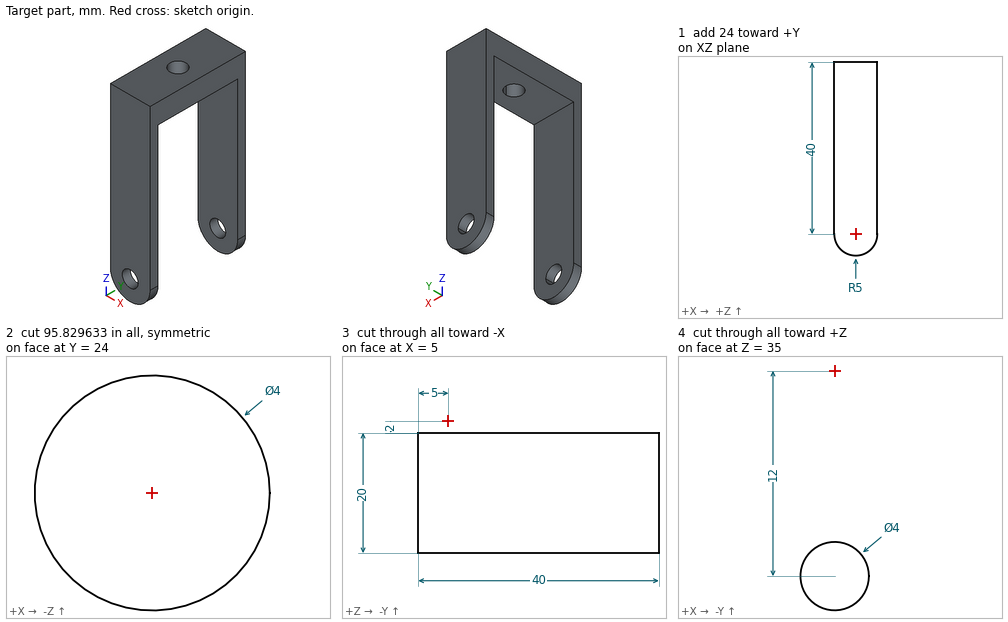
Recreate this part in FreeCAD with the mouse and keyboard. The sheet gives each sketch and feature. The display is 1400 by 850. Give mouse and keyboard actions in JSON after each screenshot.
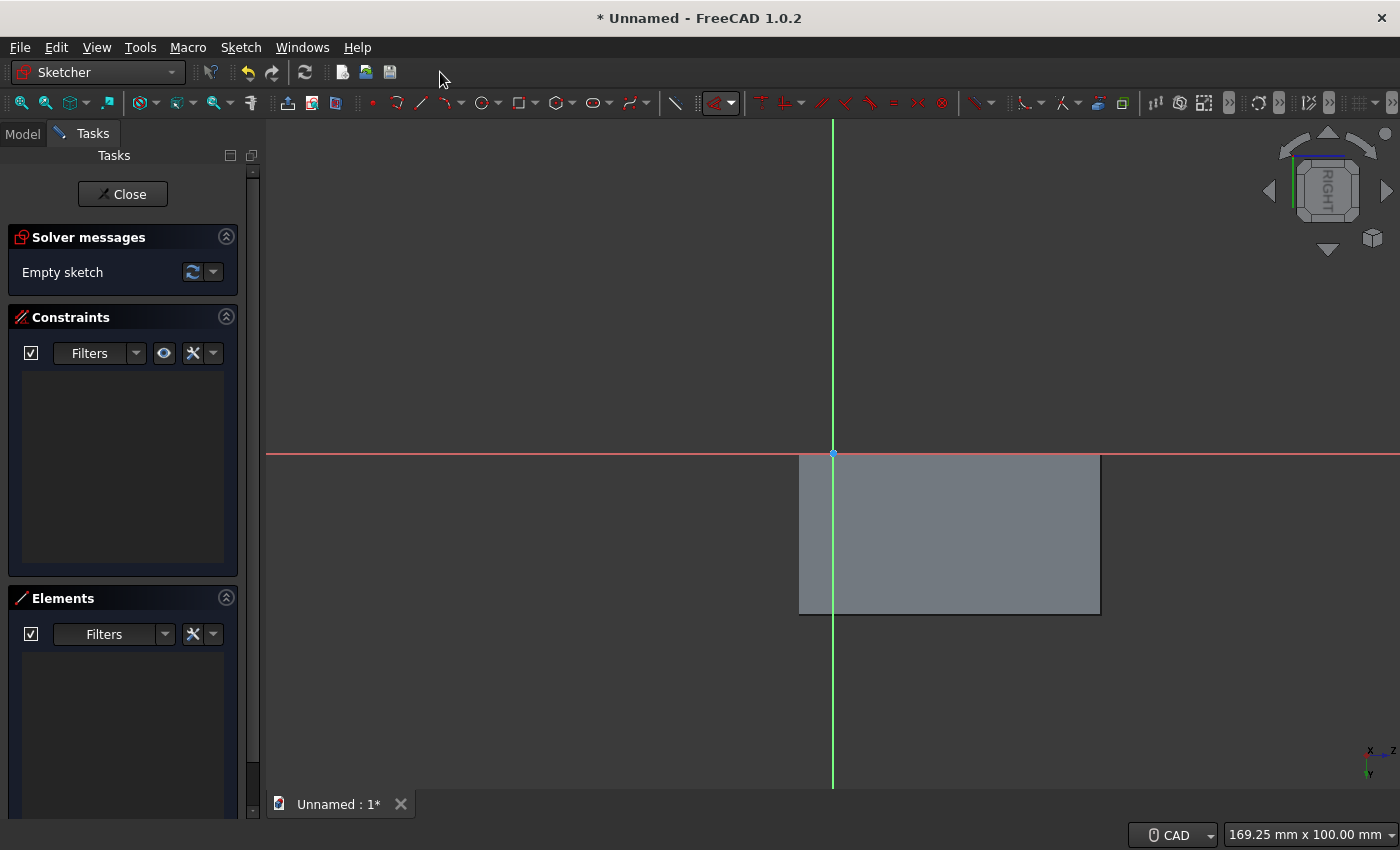
{"action": "scroll", "coordinate": [1032, 571], "scroll_direction": "up", "scroll_amount": 5}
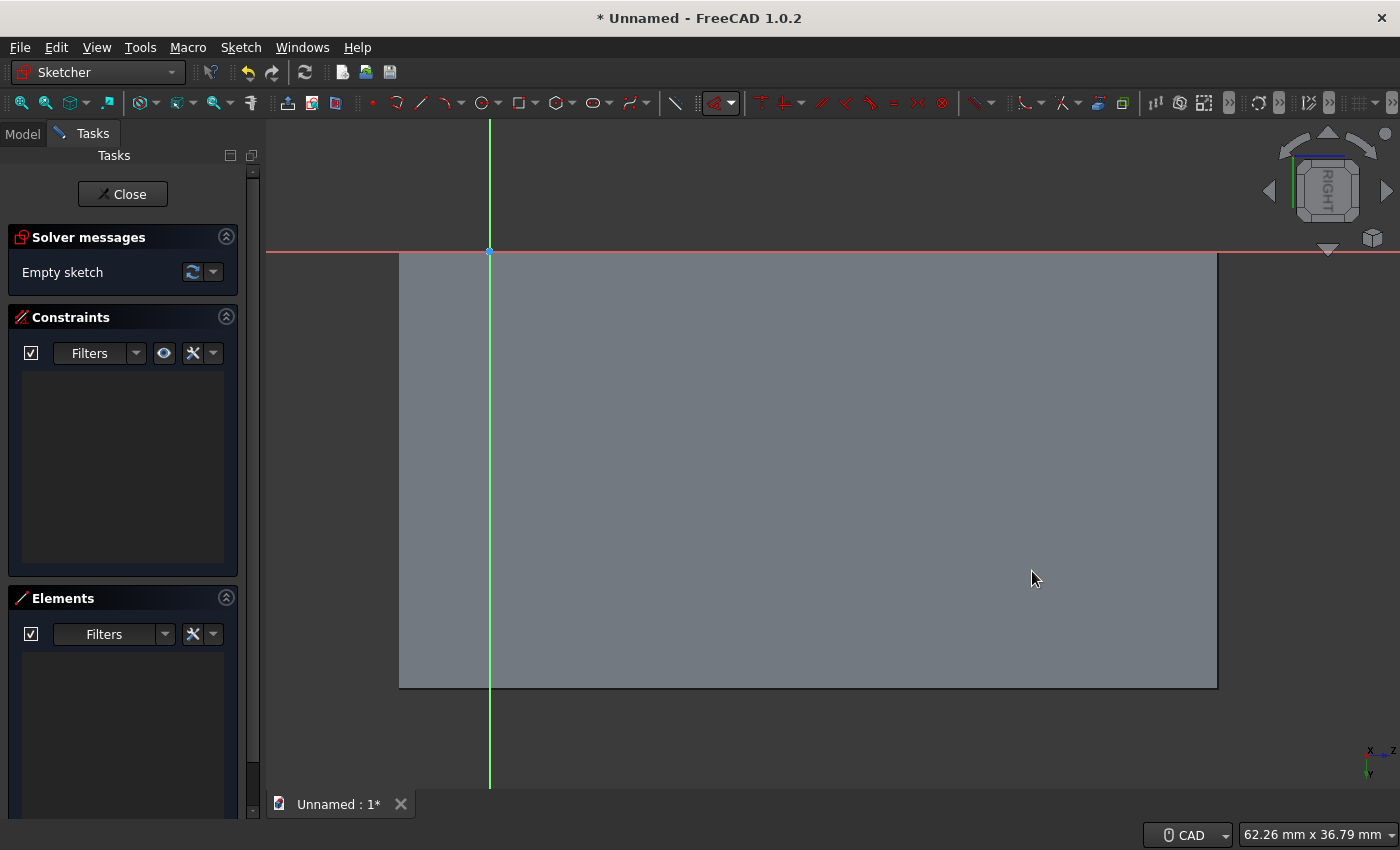
{"action": "key", "text": "g r"}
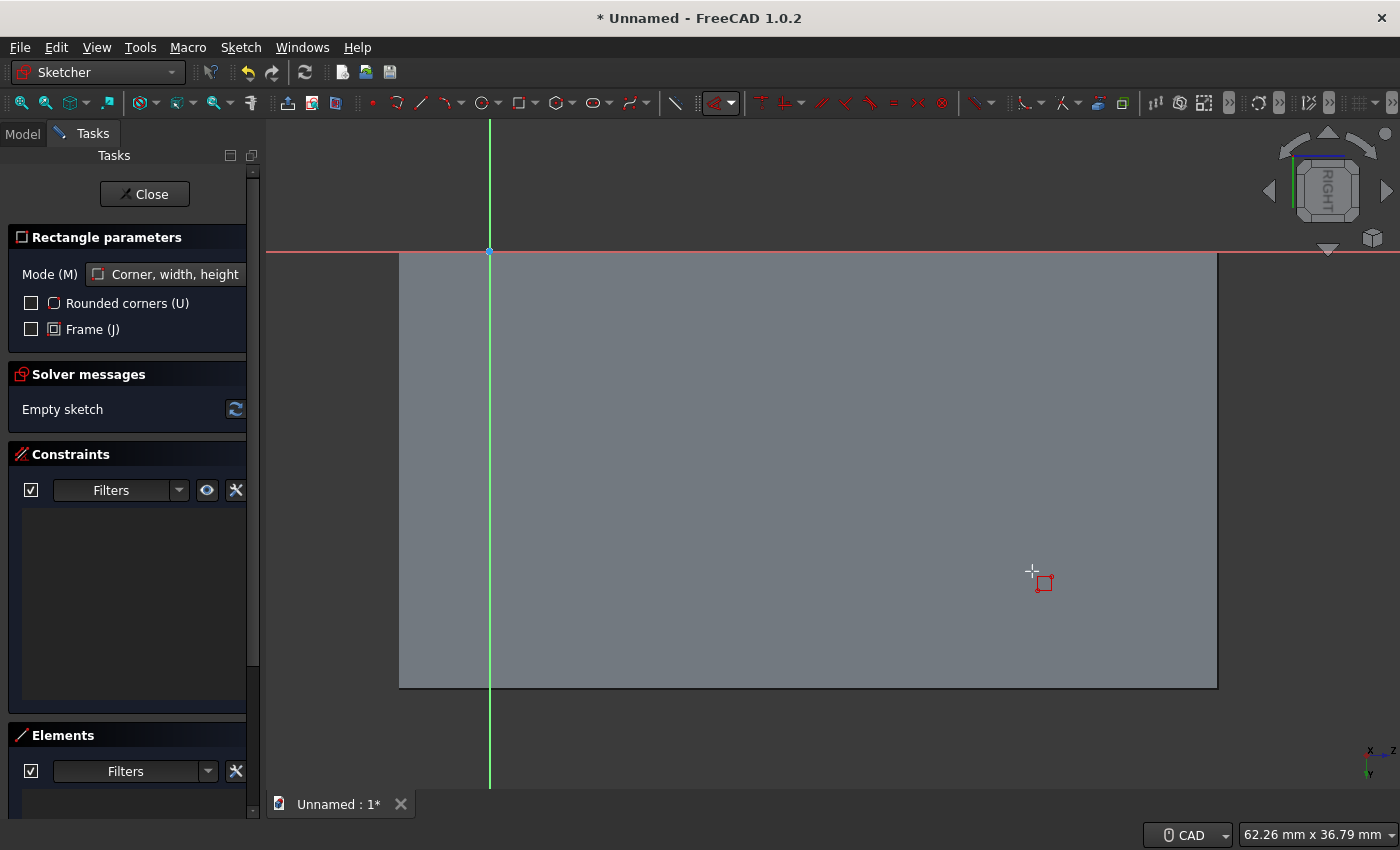
{"action": "left_click", "coordinate": [399, 288]}
{"action": "left_click", "coordinate": [1127, 652]}
{"action": "key", "text": "Escape"}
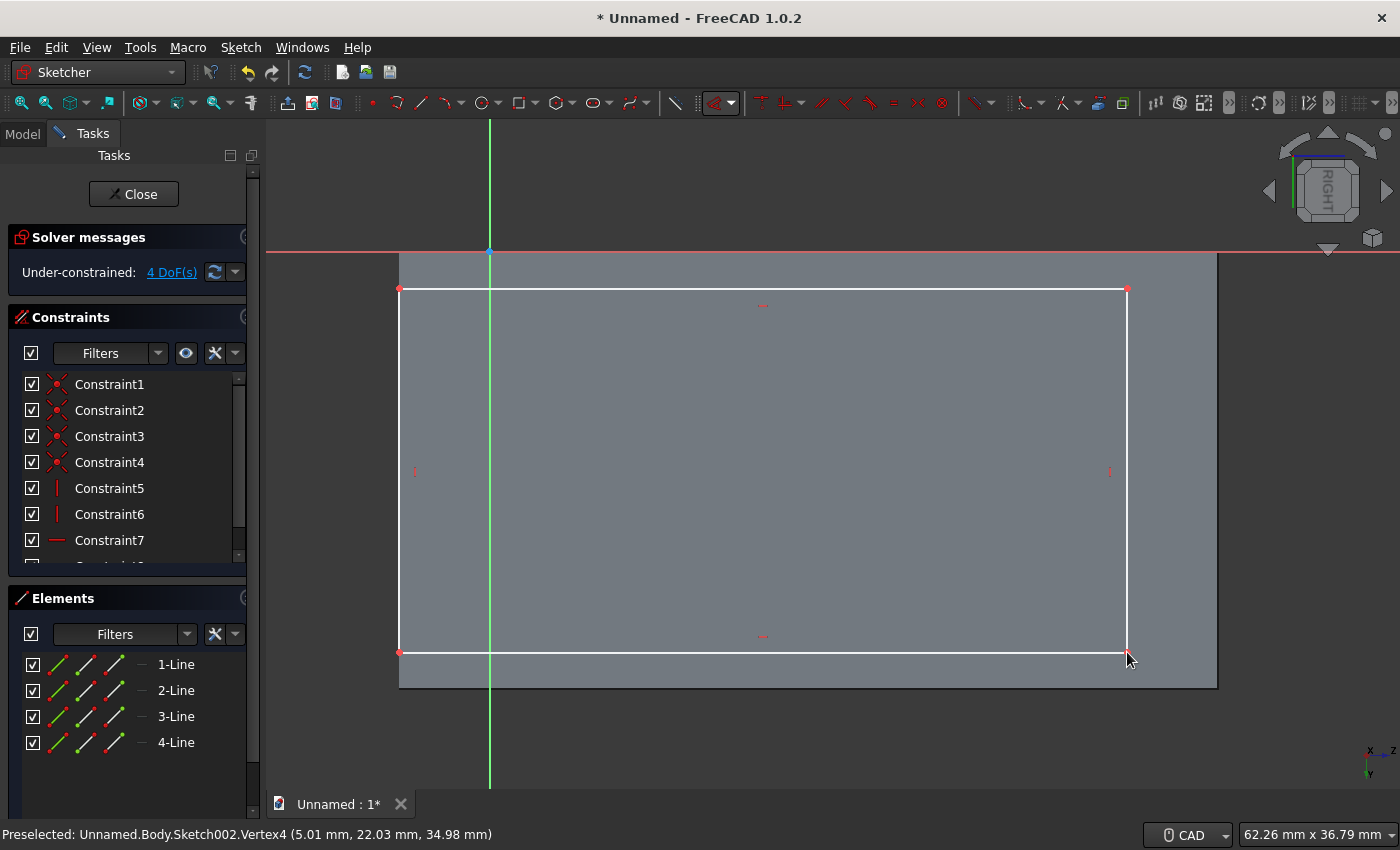
{"action": "left_click", "coordinate": [399, 398]}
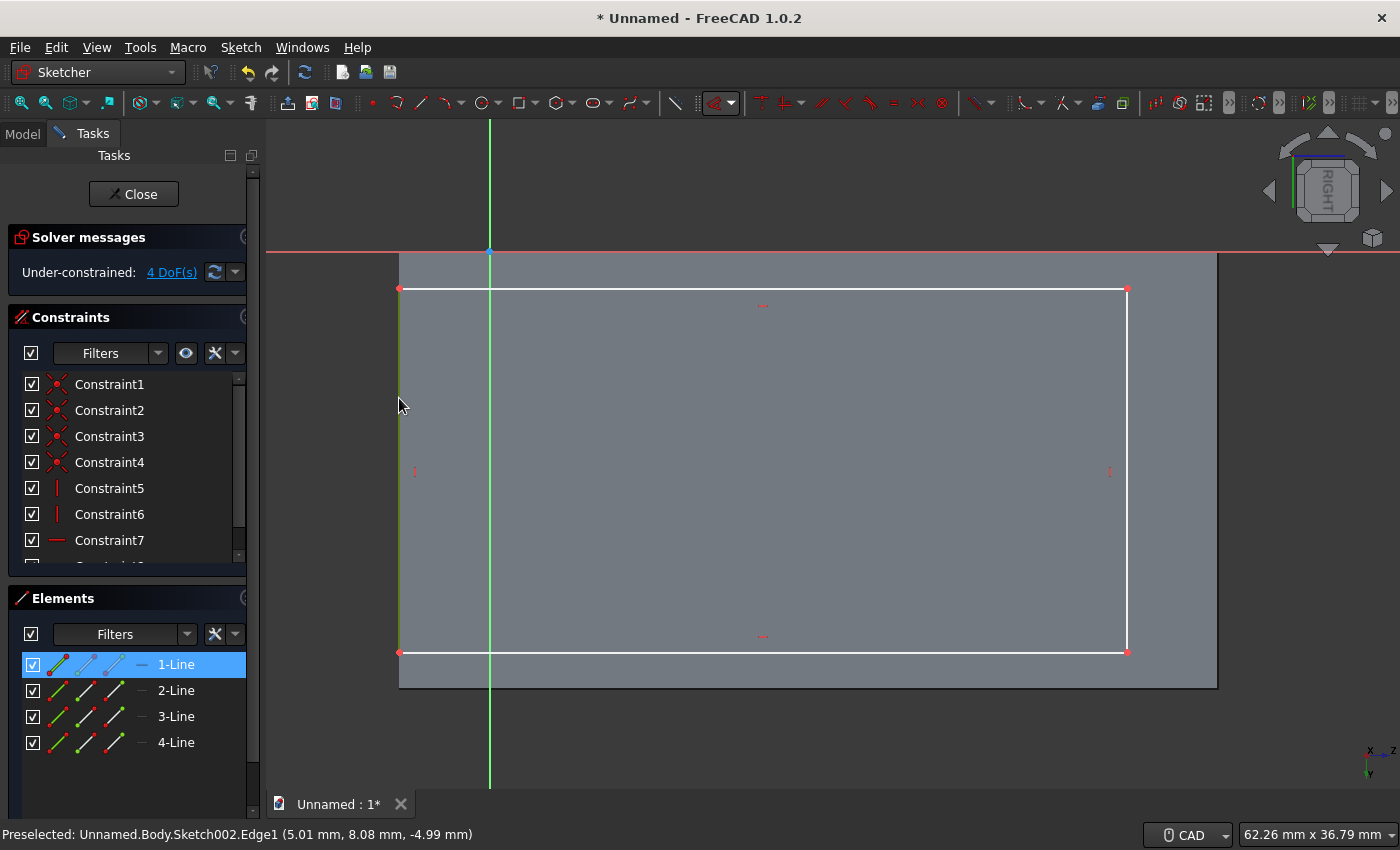
{"action": "key", "text": "i"}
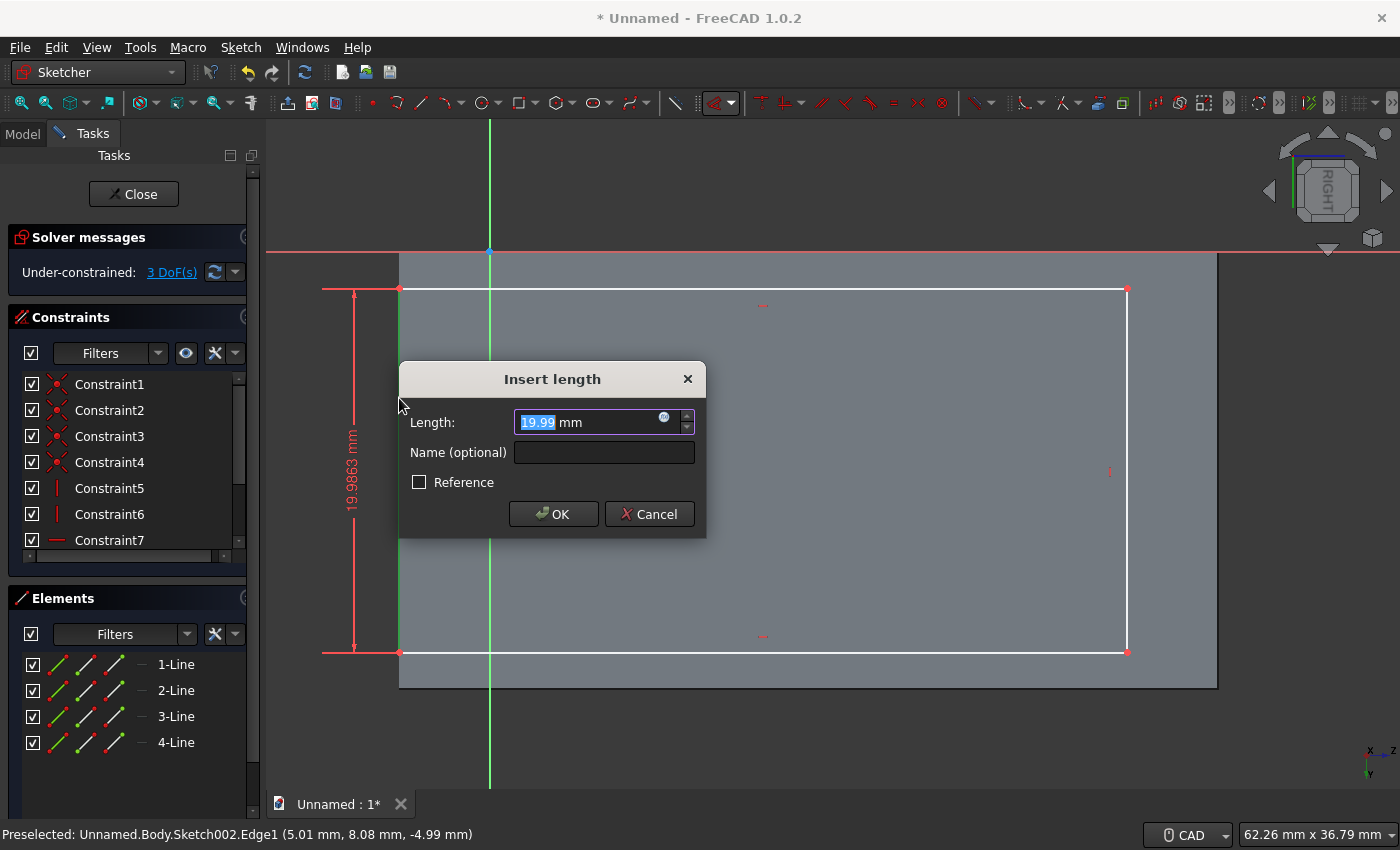
{"action": "type", "text": "20"}
{"action": "key", "text": "Return"}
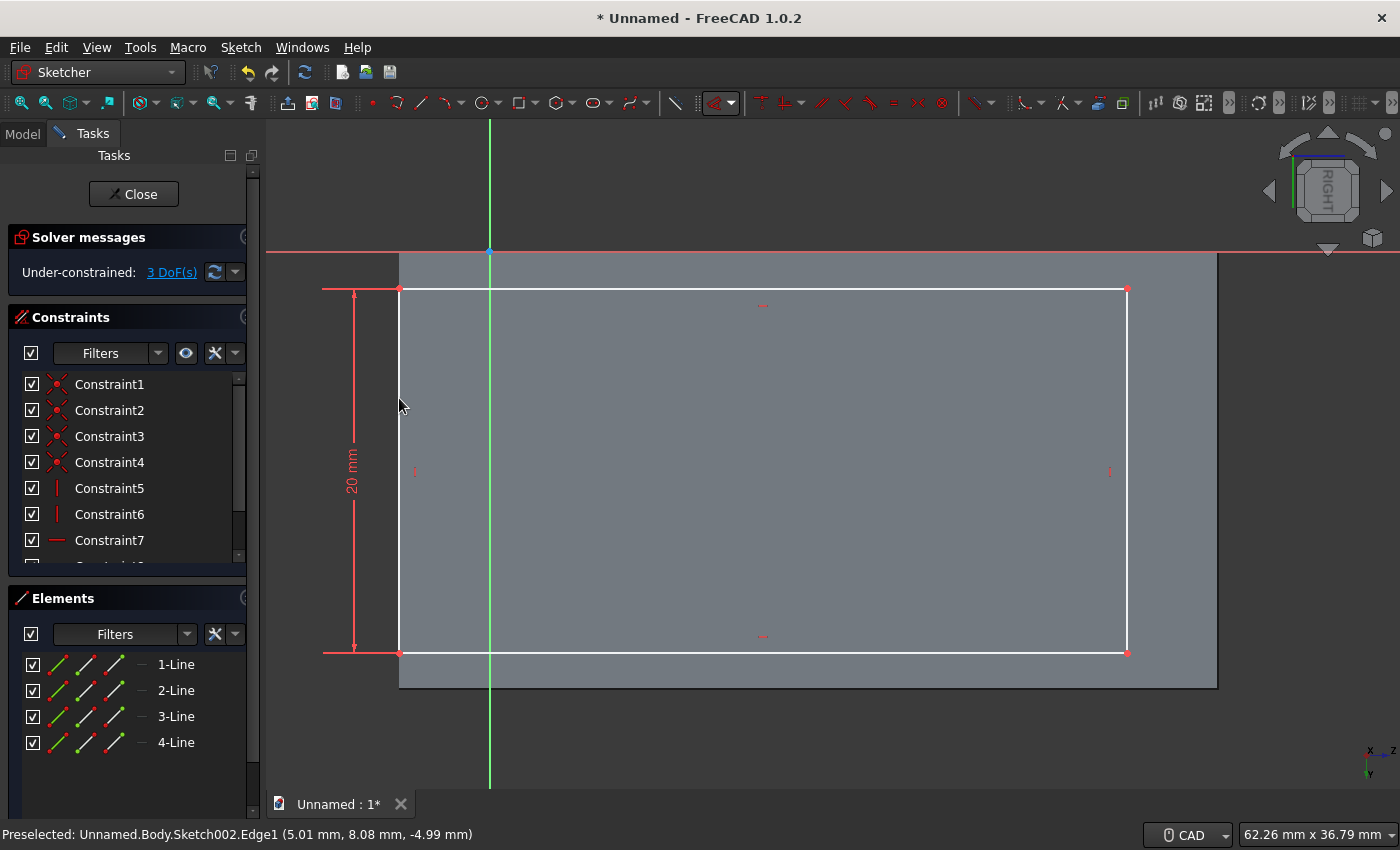
{"action": "left_click", "coordinate": [617, 653]}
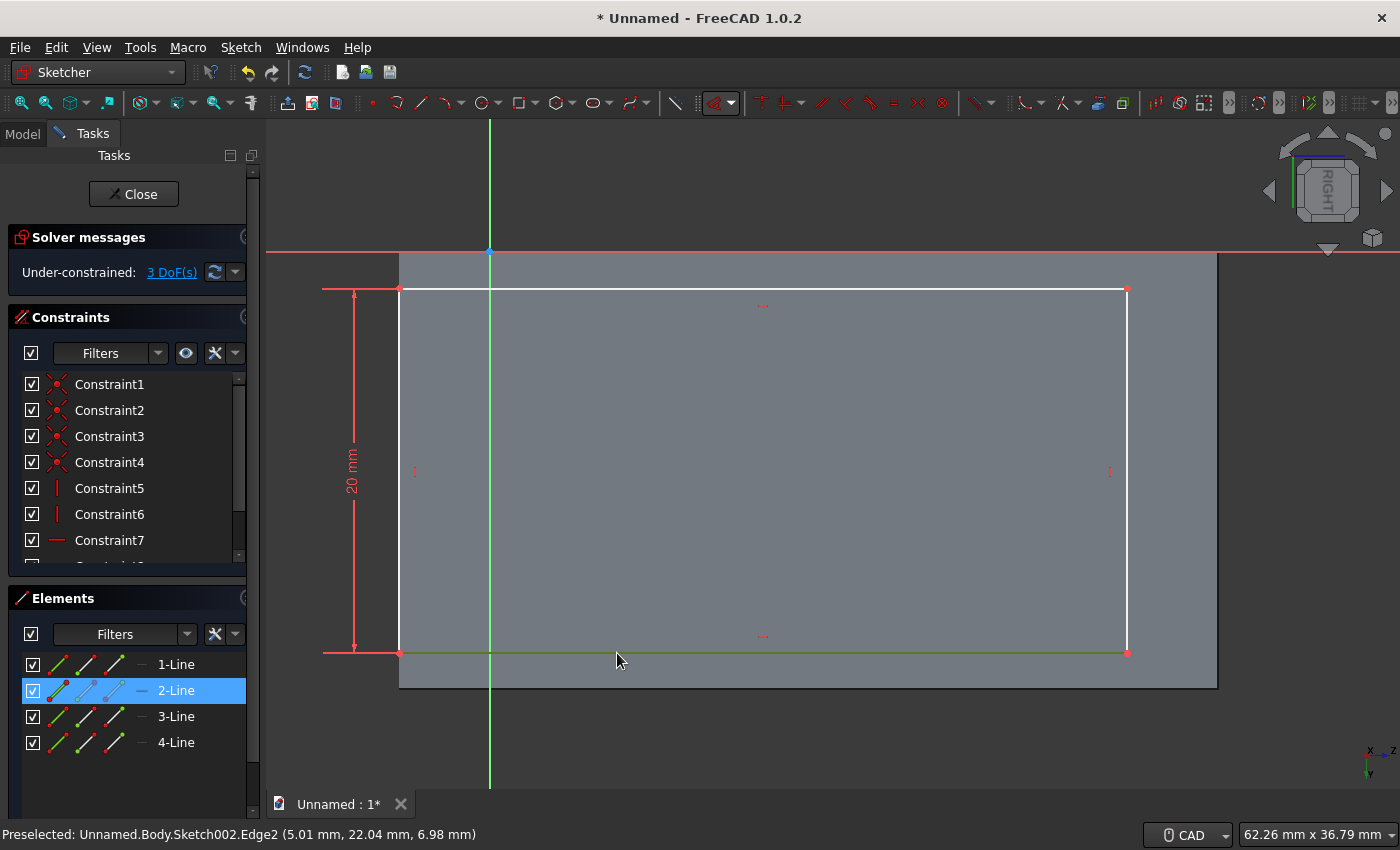
{"action": "key", "text": "l"}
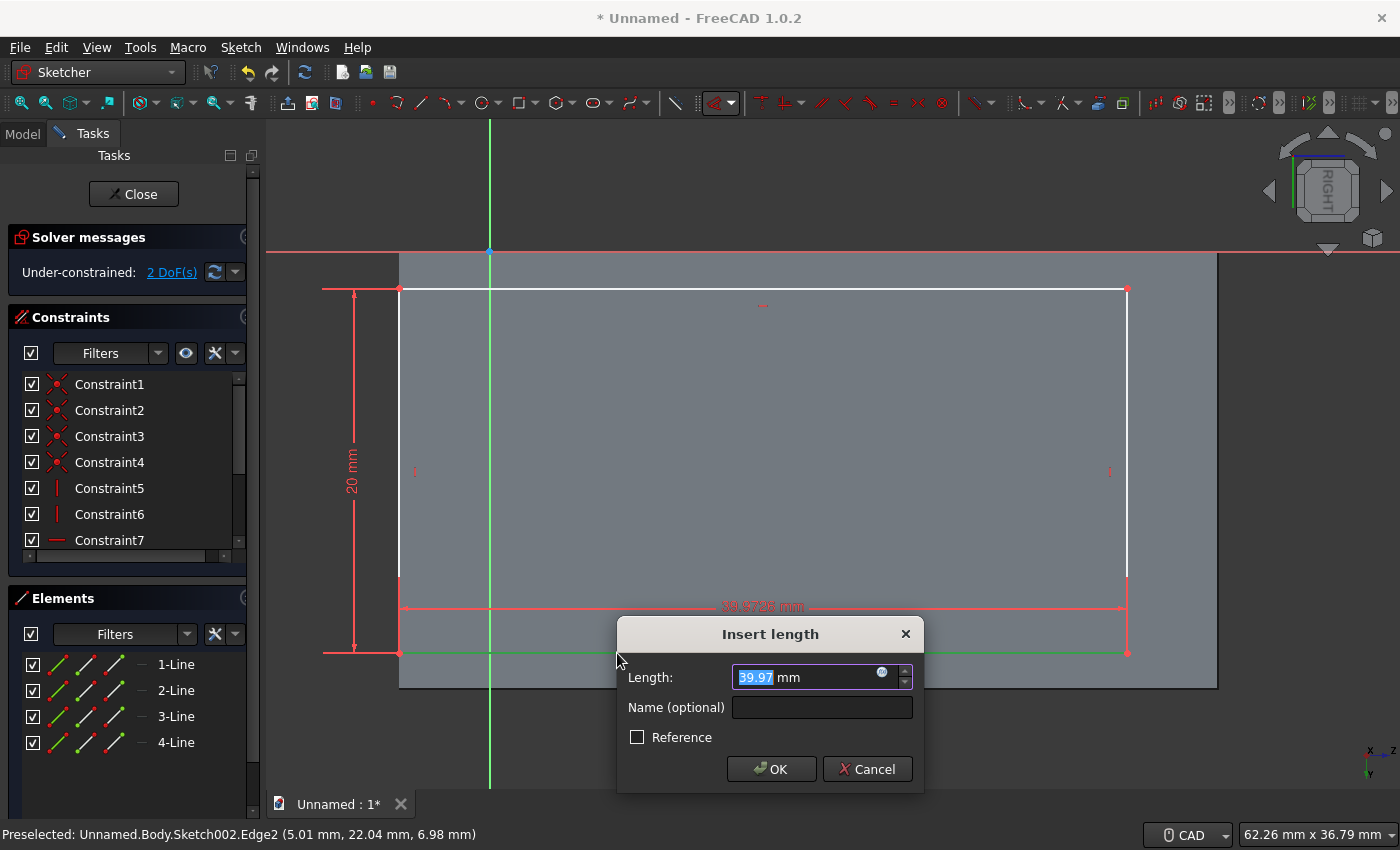
{"action": "type", "text": "40"}
{"action": "key", "text": "Return"}